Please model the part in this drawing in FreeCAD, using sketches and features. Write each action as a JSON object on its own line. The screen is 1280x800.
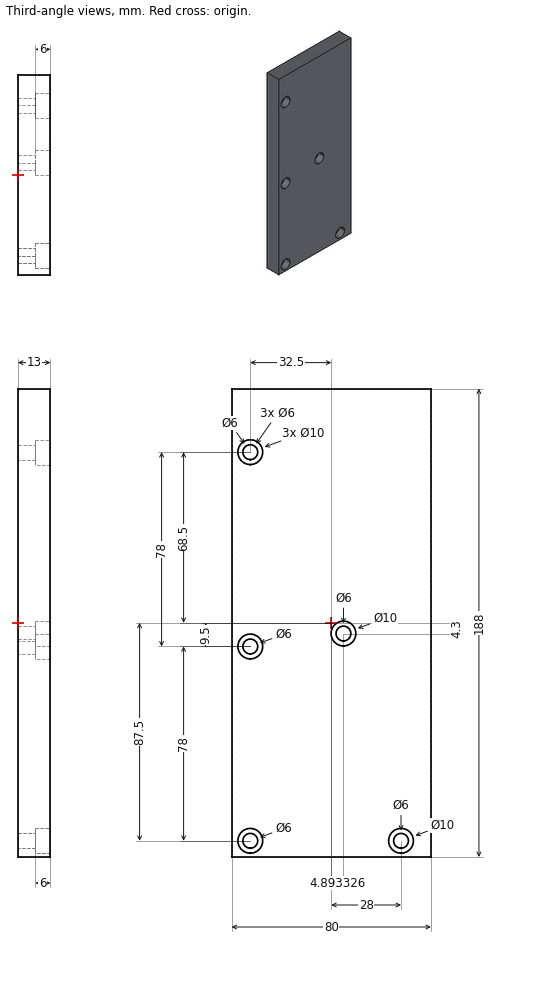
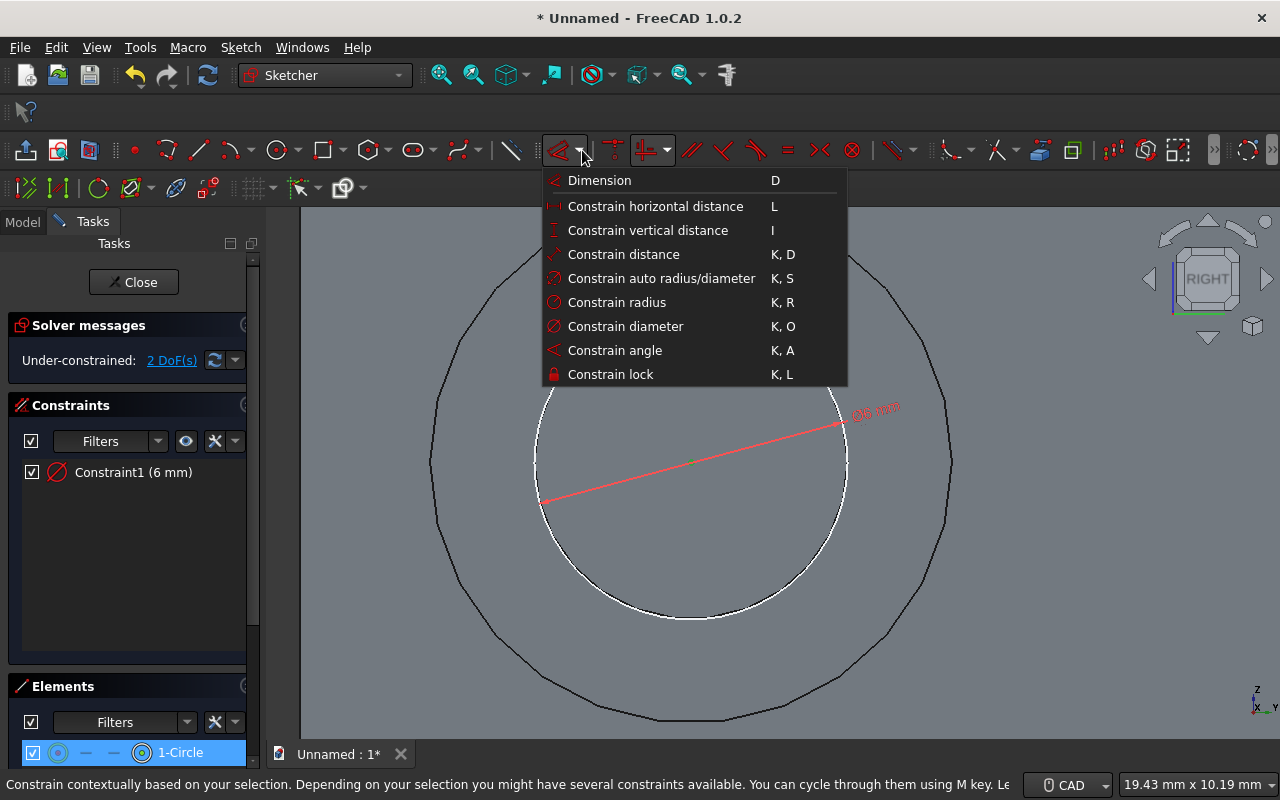
{"action": "left_click", "coordinate": [695, 230]}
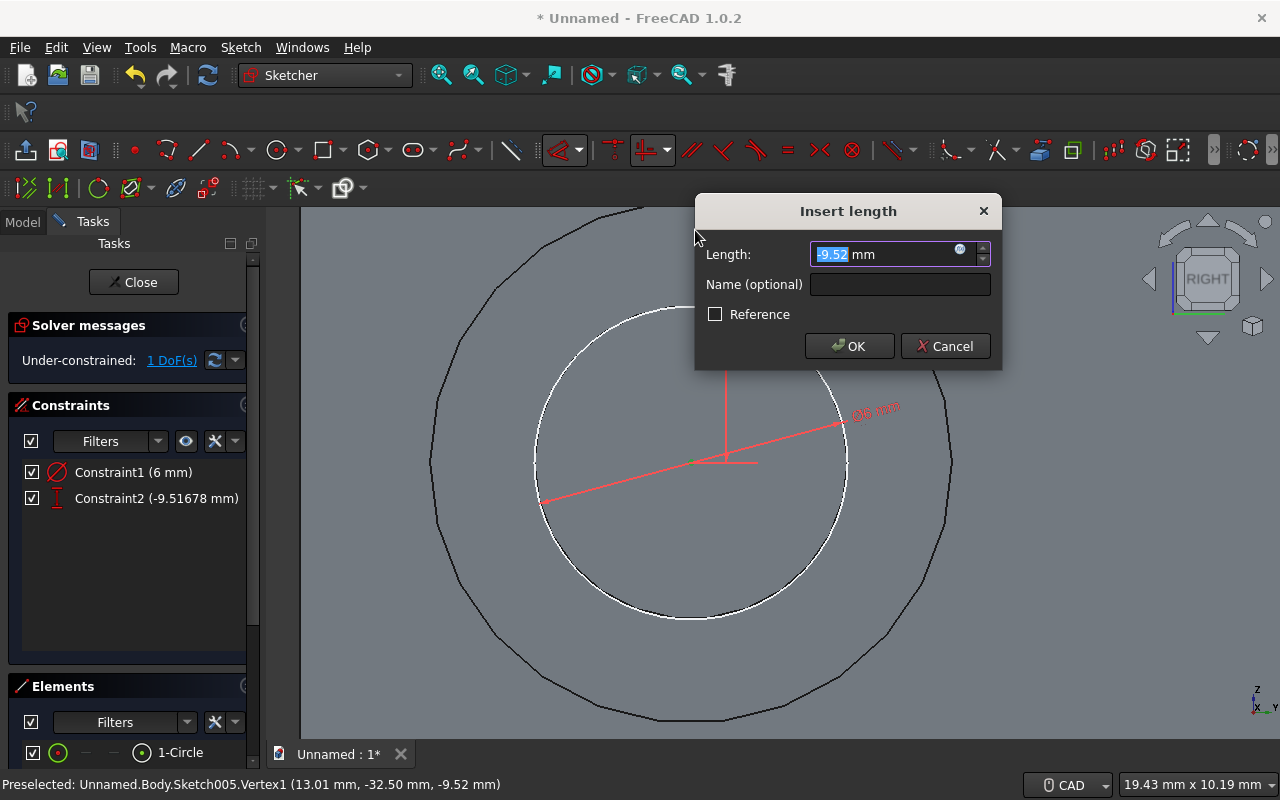
{"action": "type", "text": "-9.5"}
{"action": "key", "text": "Return"}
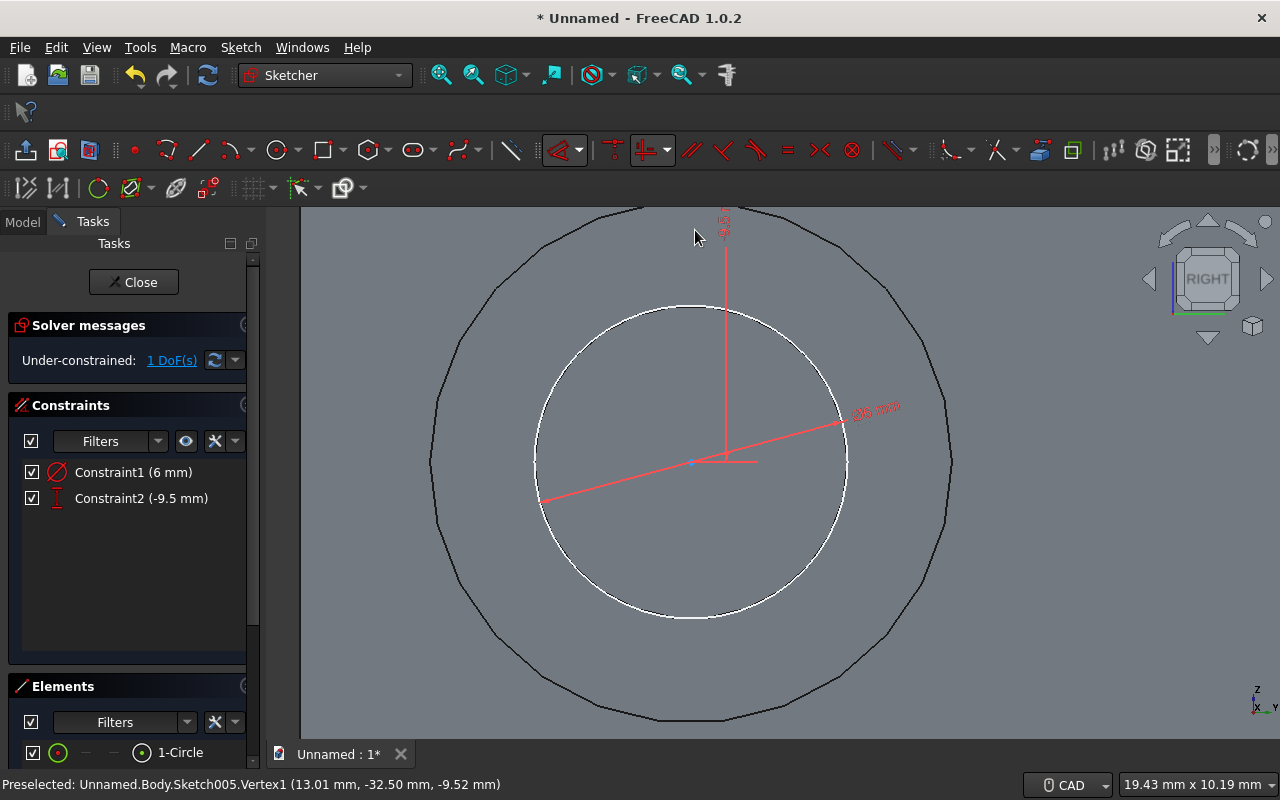
{"action": "left_click", "coordinate": [691, 462]}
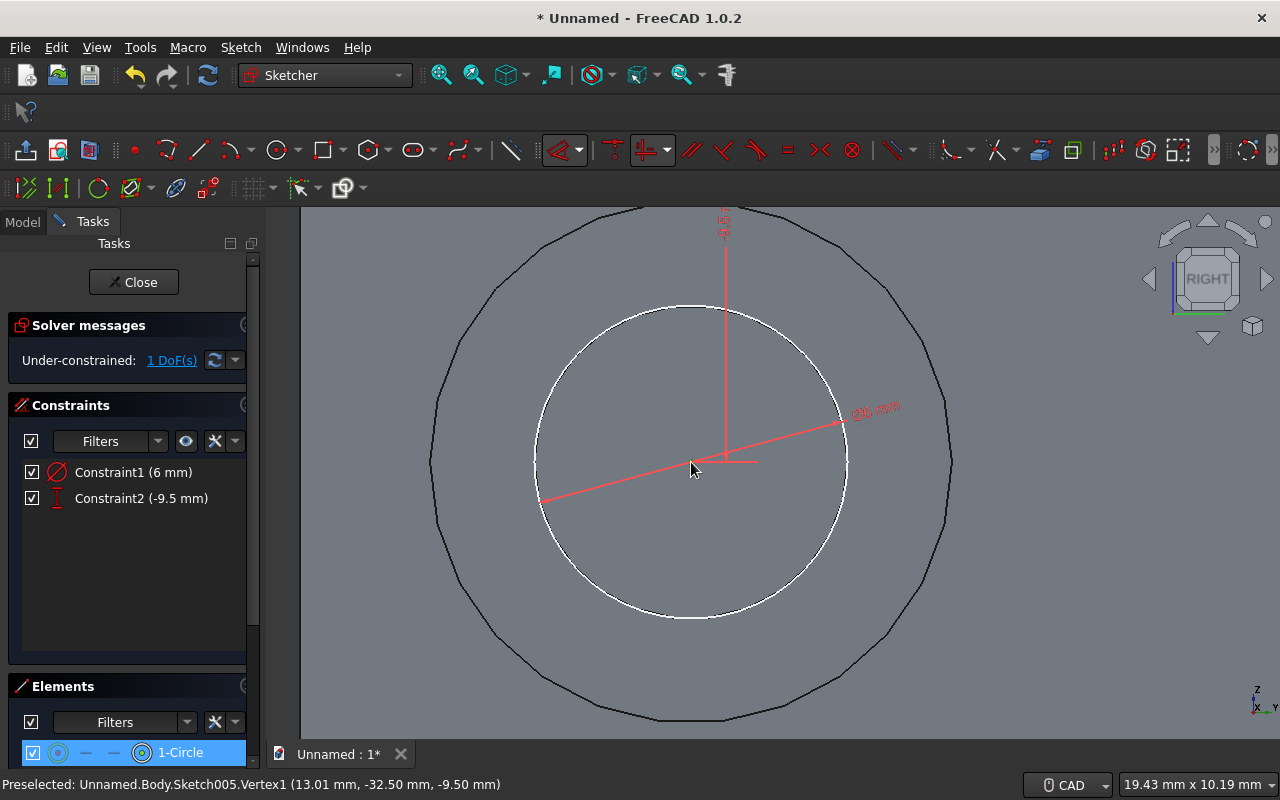
{"action": "left_click", "coordinate": [582, 150]}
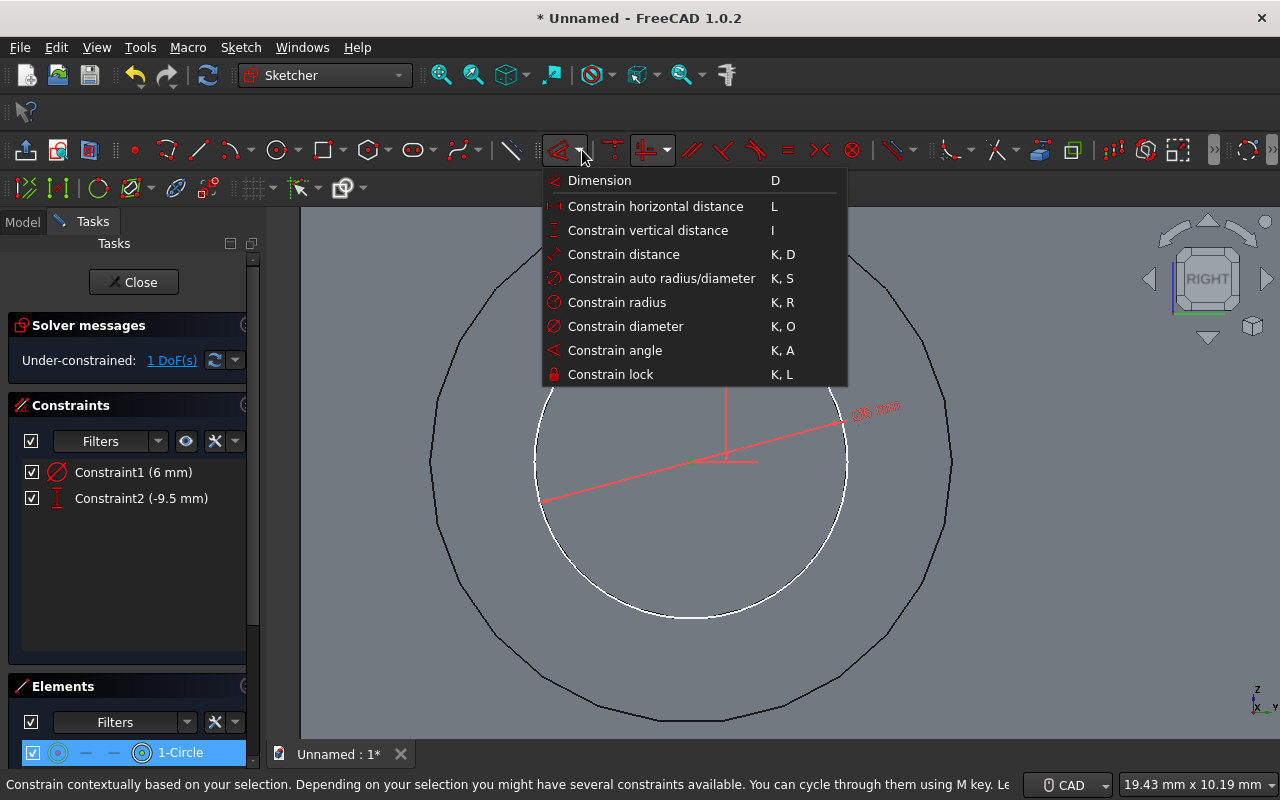
{"action": "left_click", "coordinate": [695, 206]}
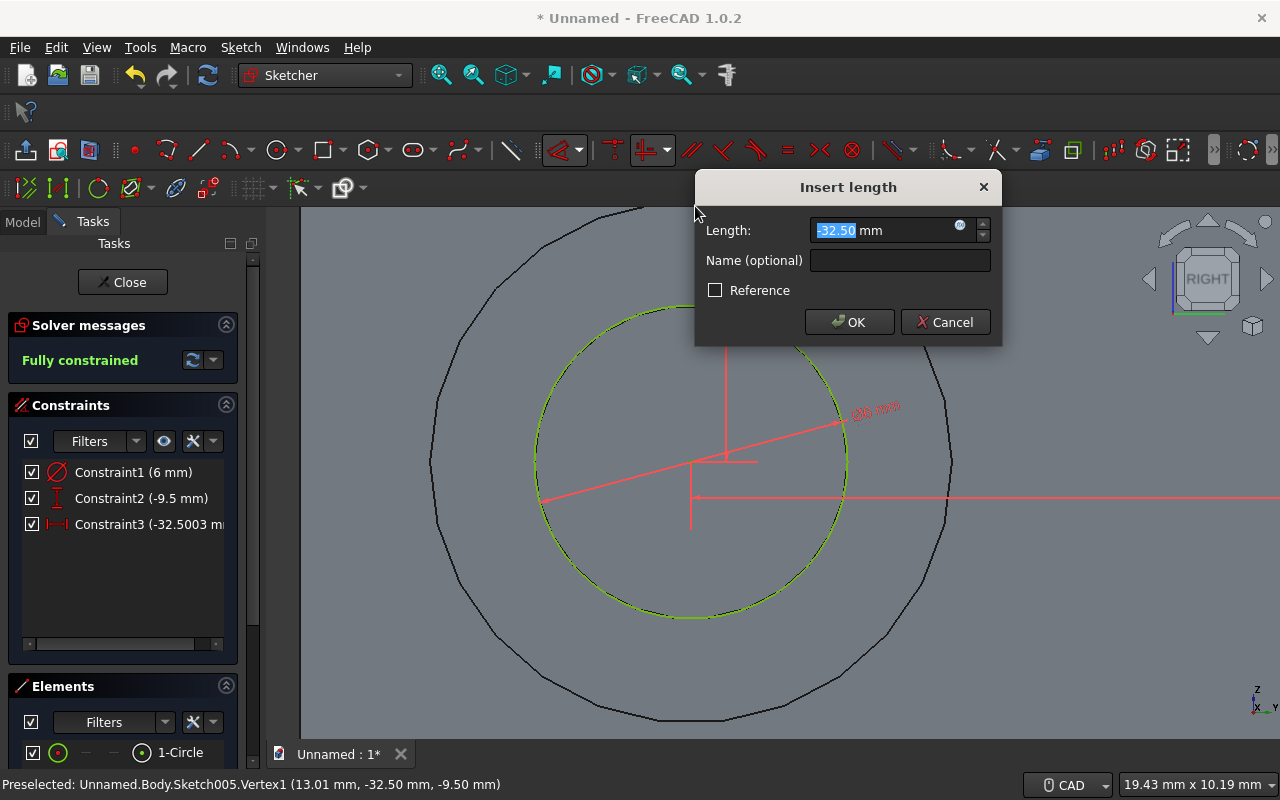
{"action": "type", "text": "-32.5"}
{"action": "key", "text": "Return"}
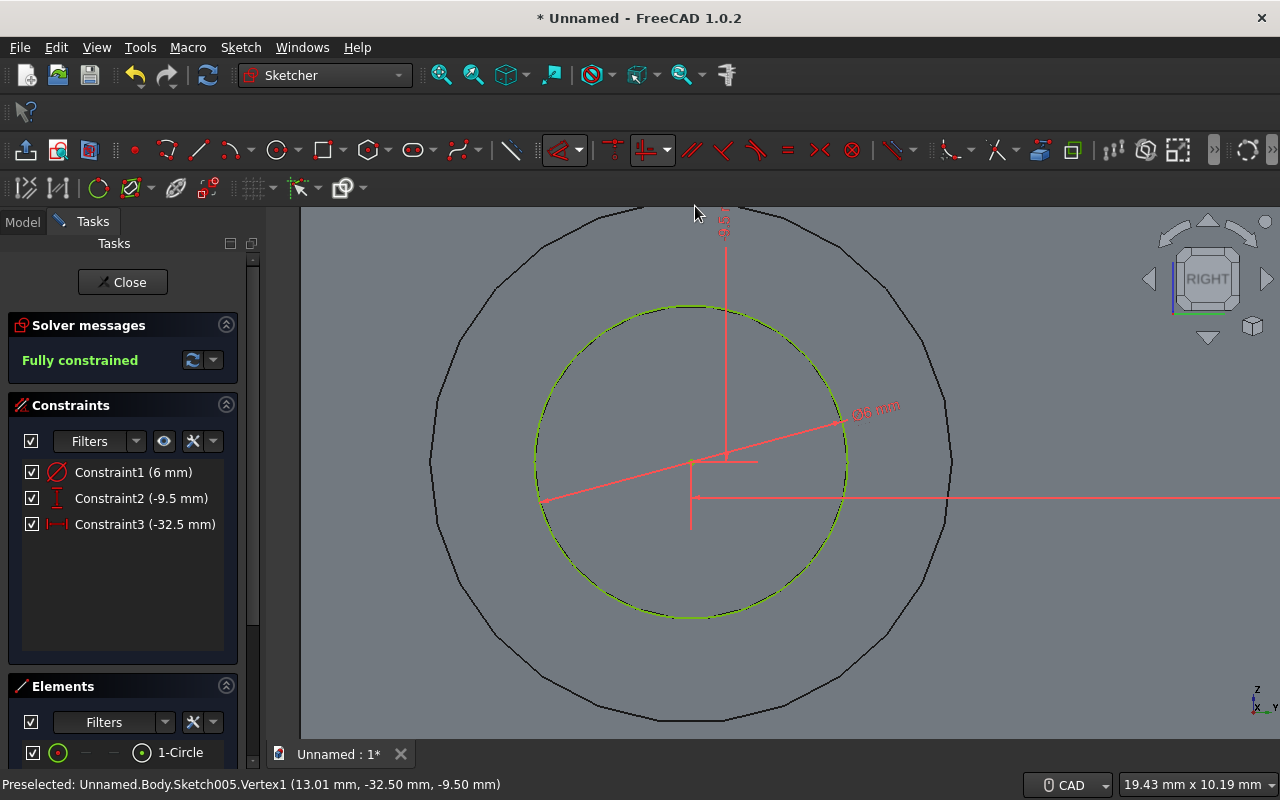
{"action": "left_click", "coordinate": [123, 282]}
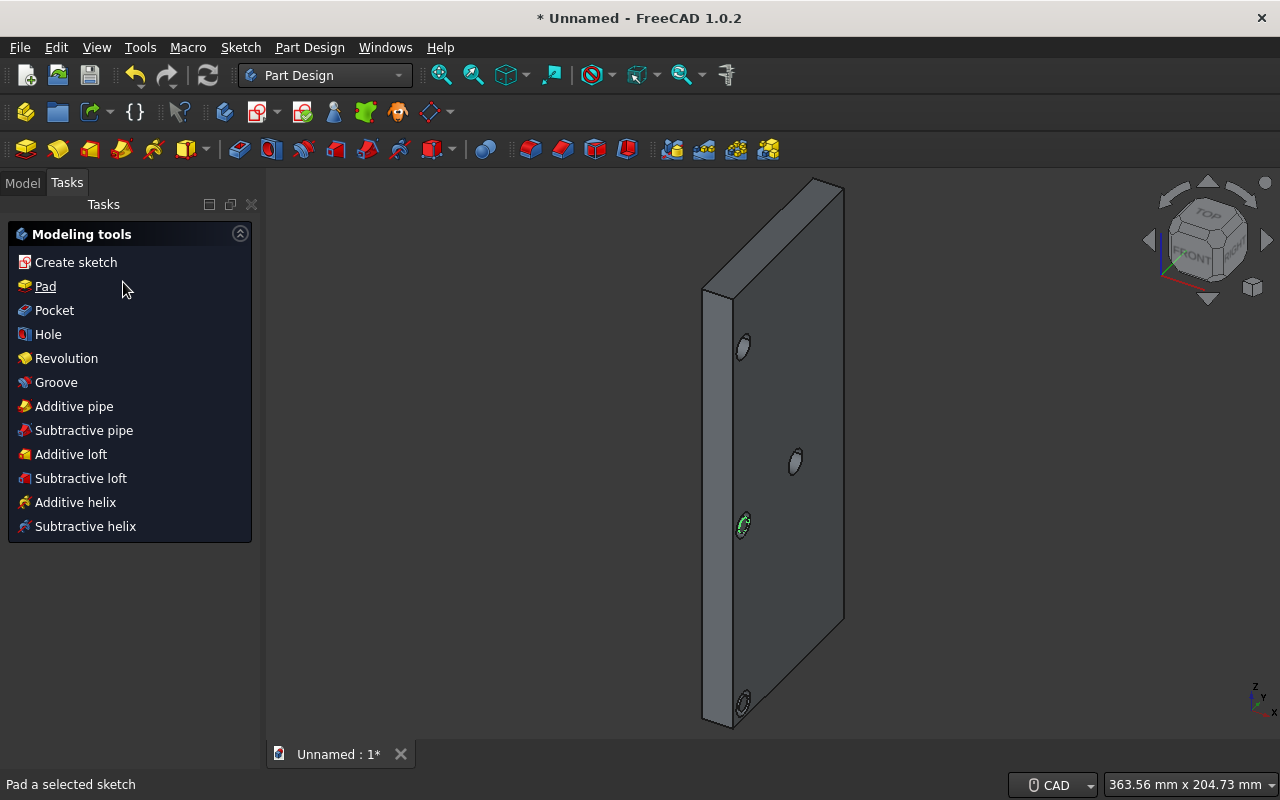
{"action": "left_click", "coordinate": [240, 150]}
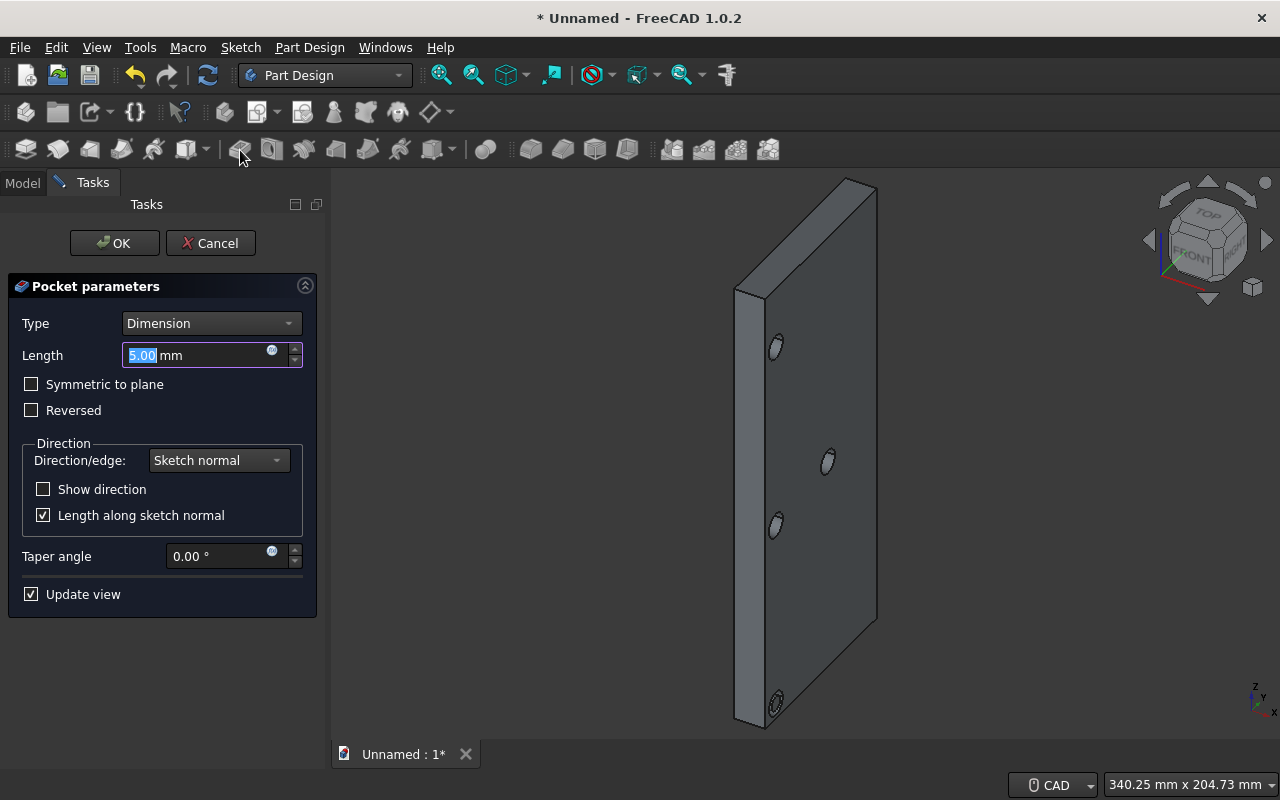
{"action": "left_click", "coordinate": [212, 324]}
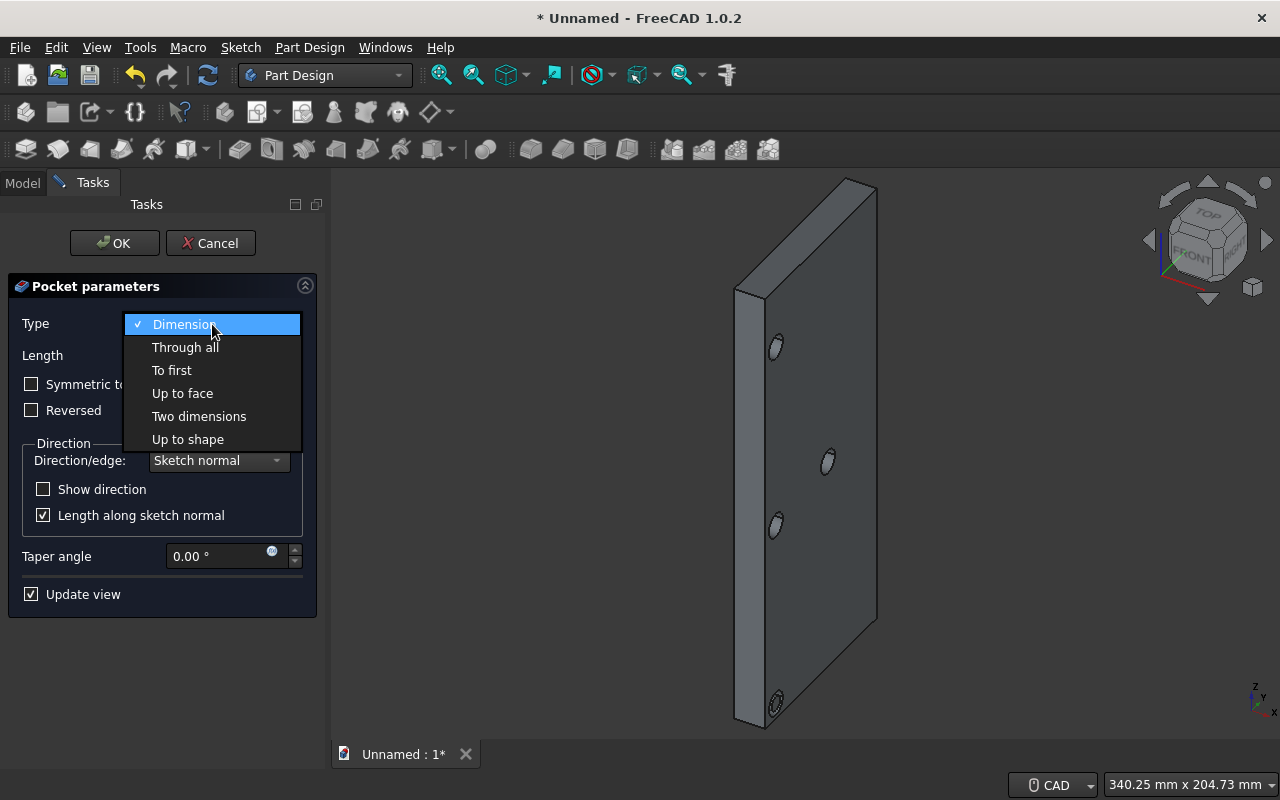
{"action": "left_click", "coordinate": [212, 370]}